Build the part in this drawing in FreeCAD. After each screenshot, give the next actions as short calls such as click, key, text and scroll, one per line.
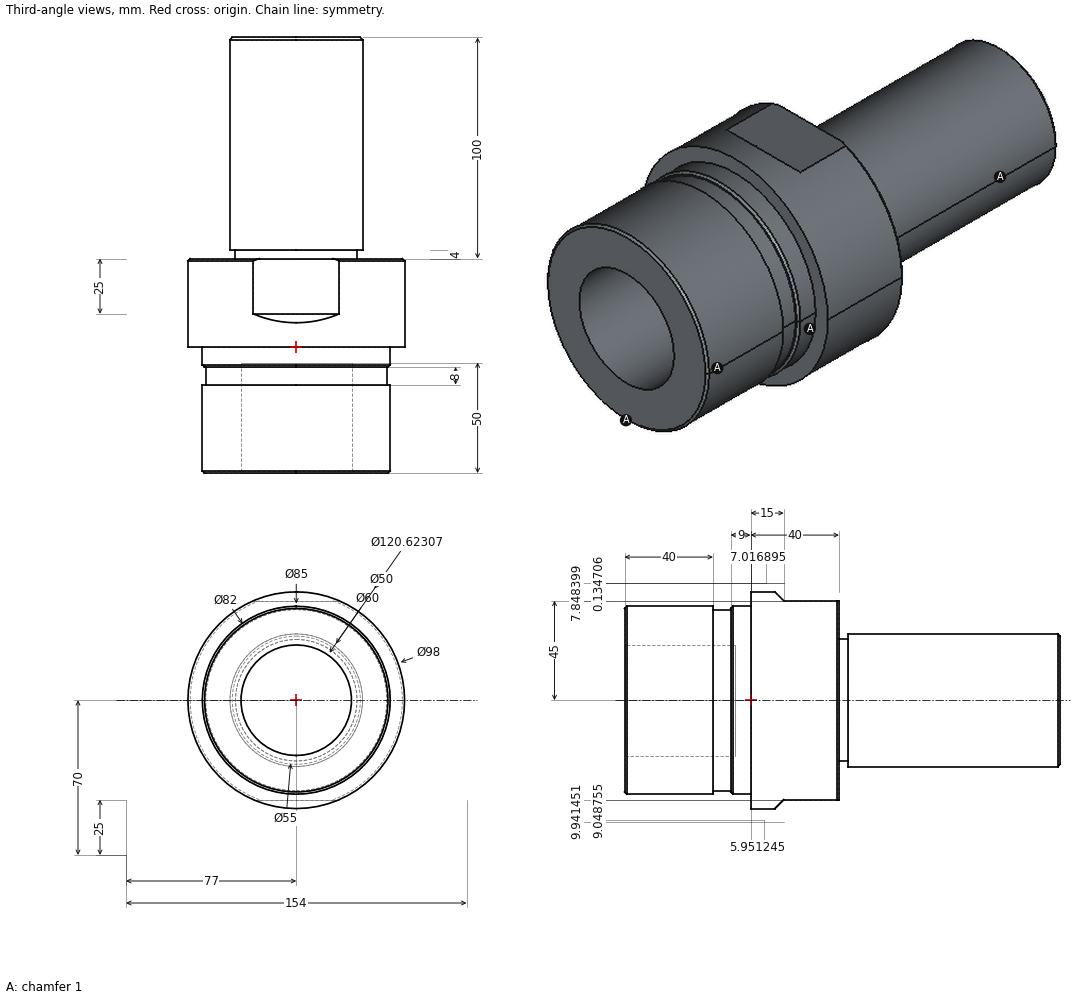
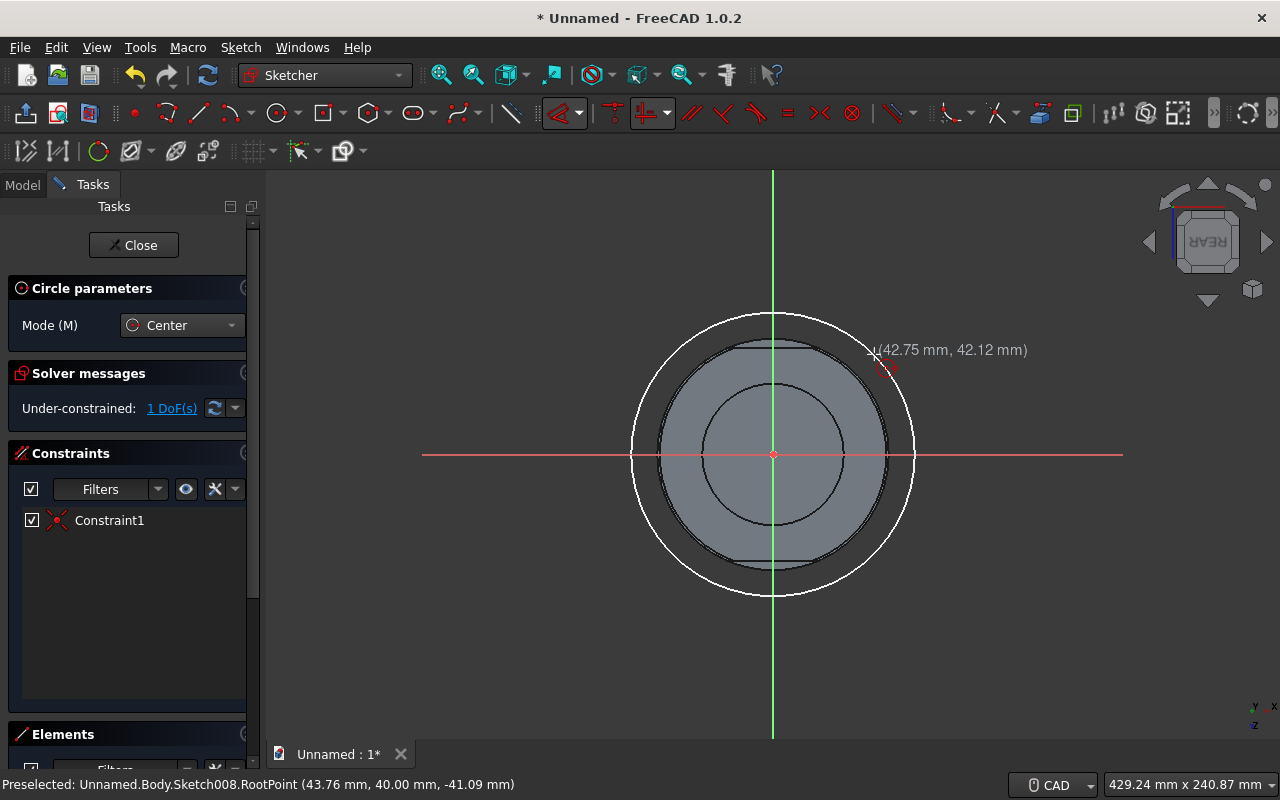
click(773, 454)
click(819, 409)
key(Escape)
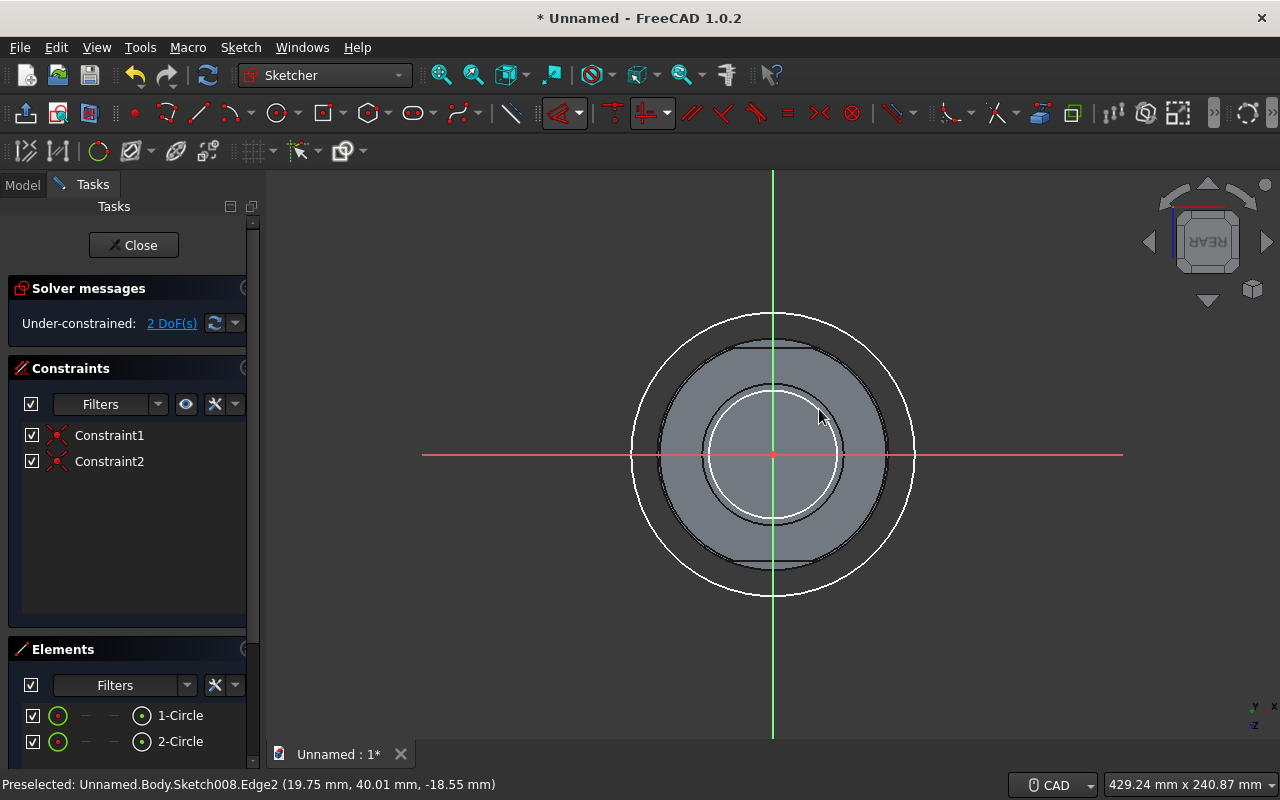
click(873, 354)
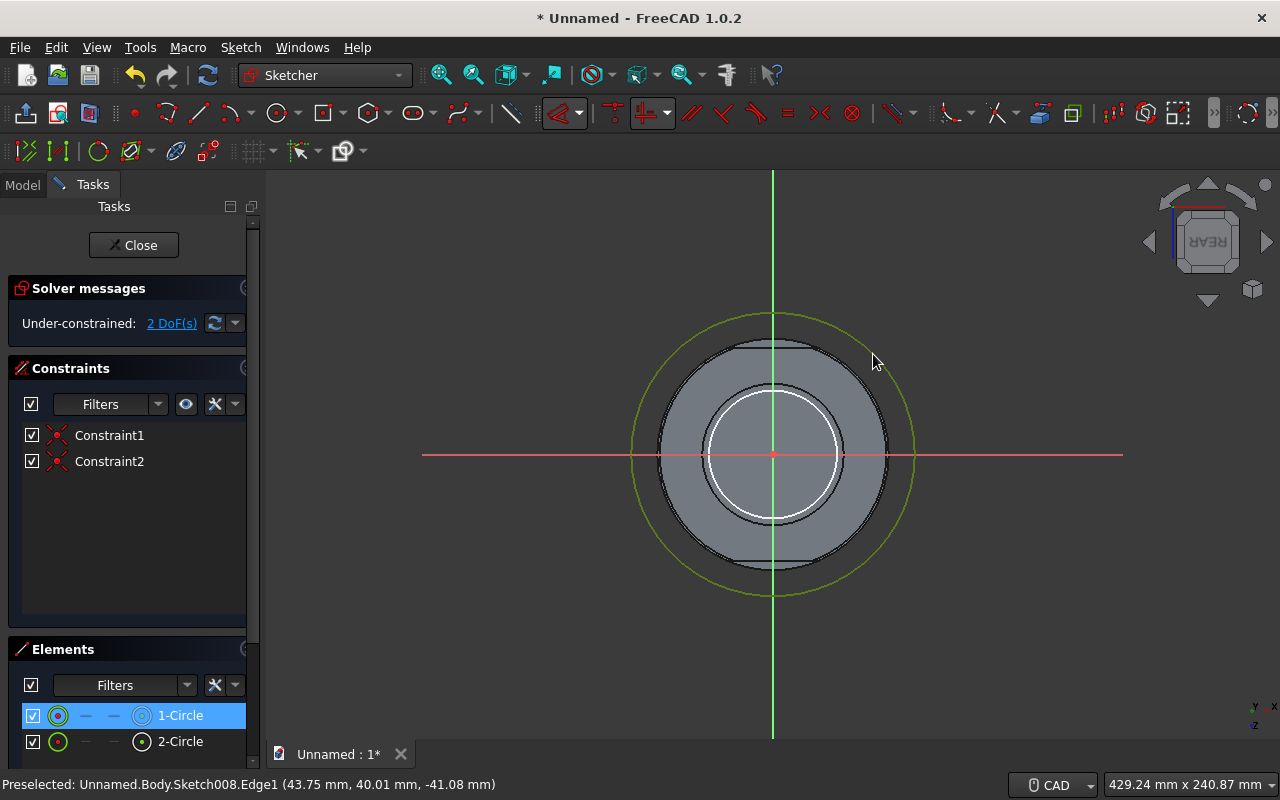
click(582, 114)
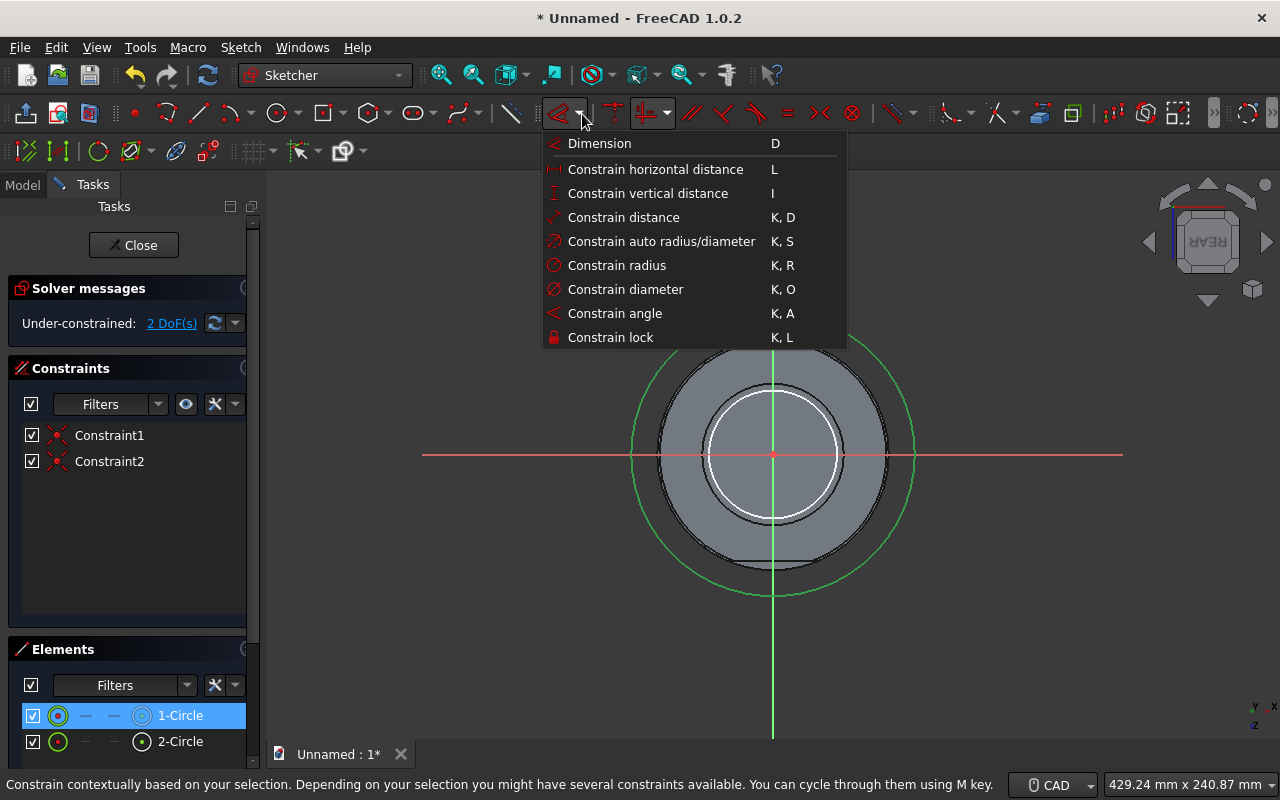
click(695, 289)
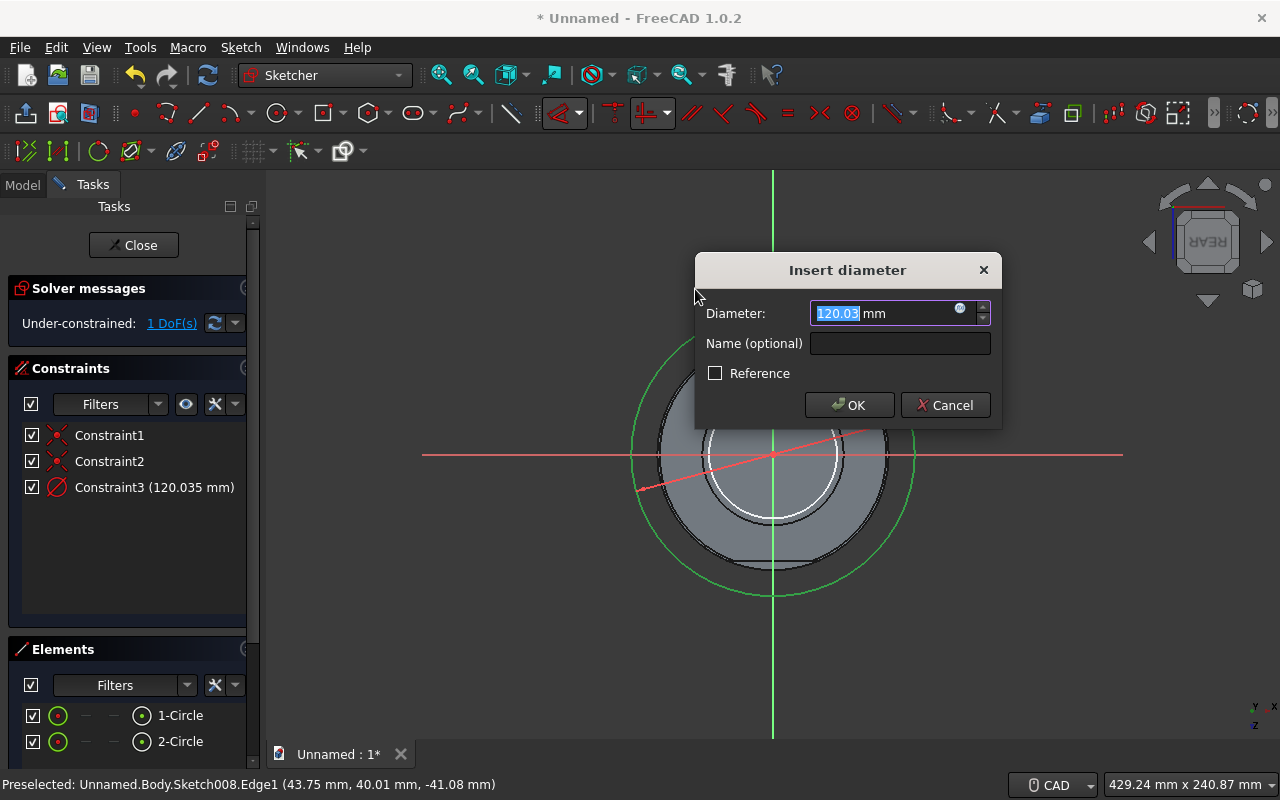
text(120.62307)
key(Return)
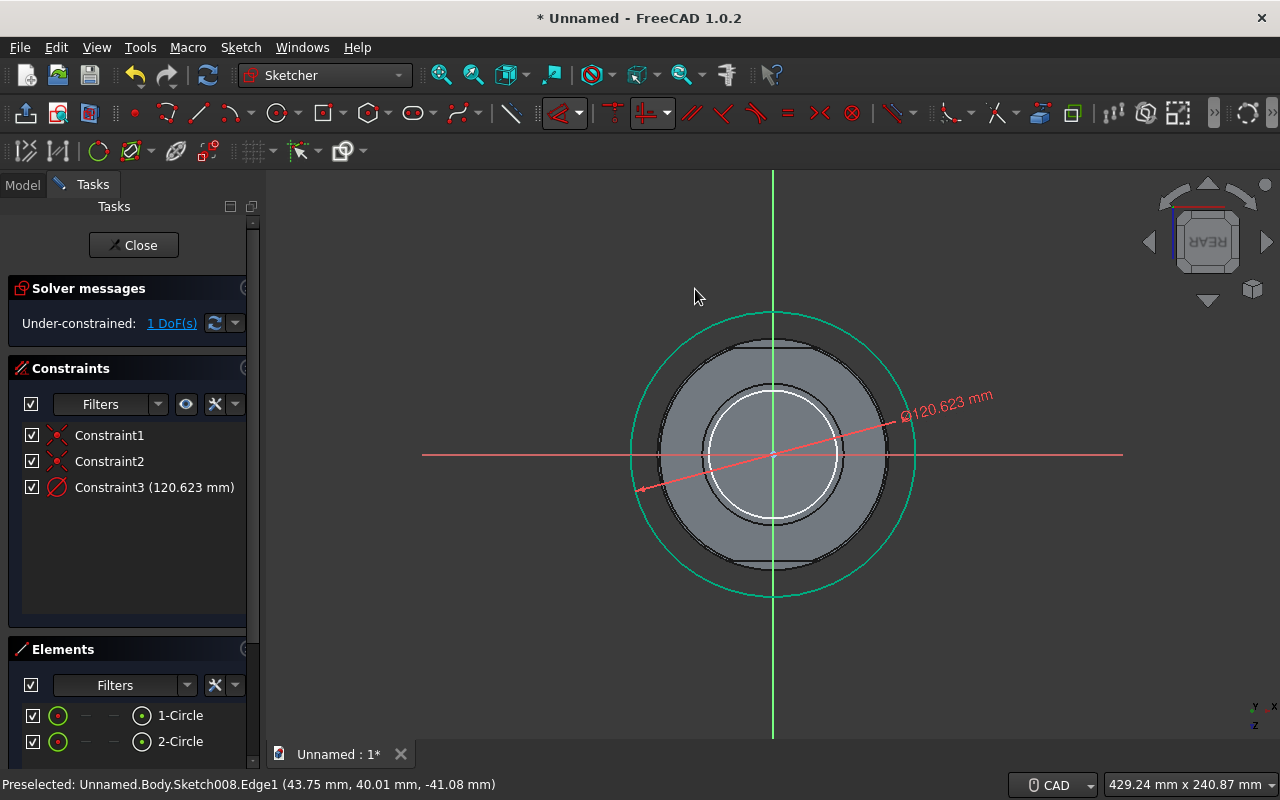
click(818, 409)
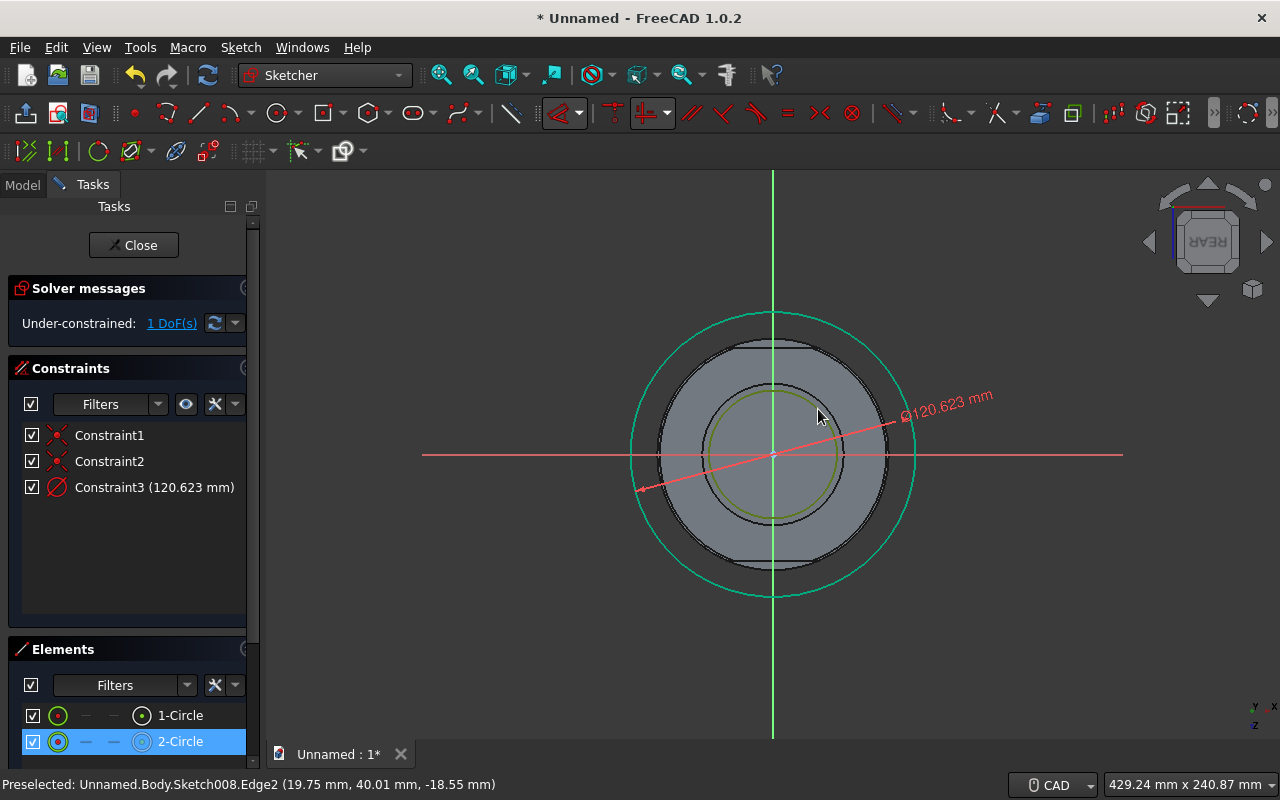
click(582, 114)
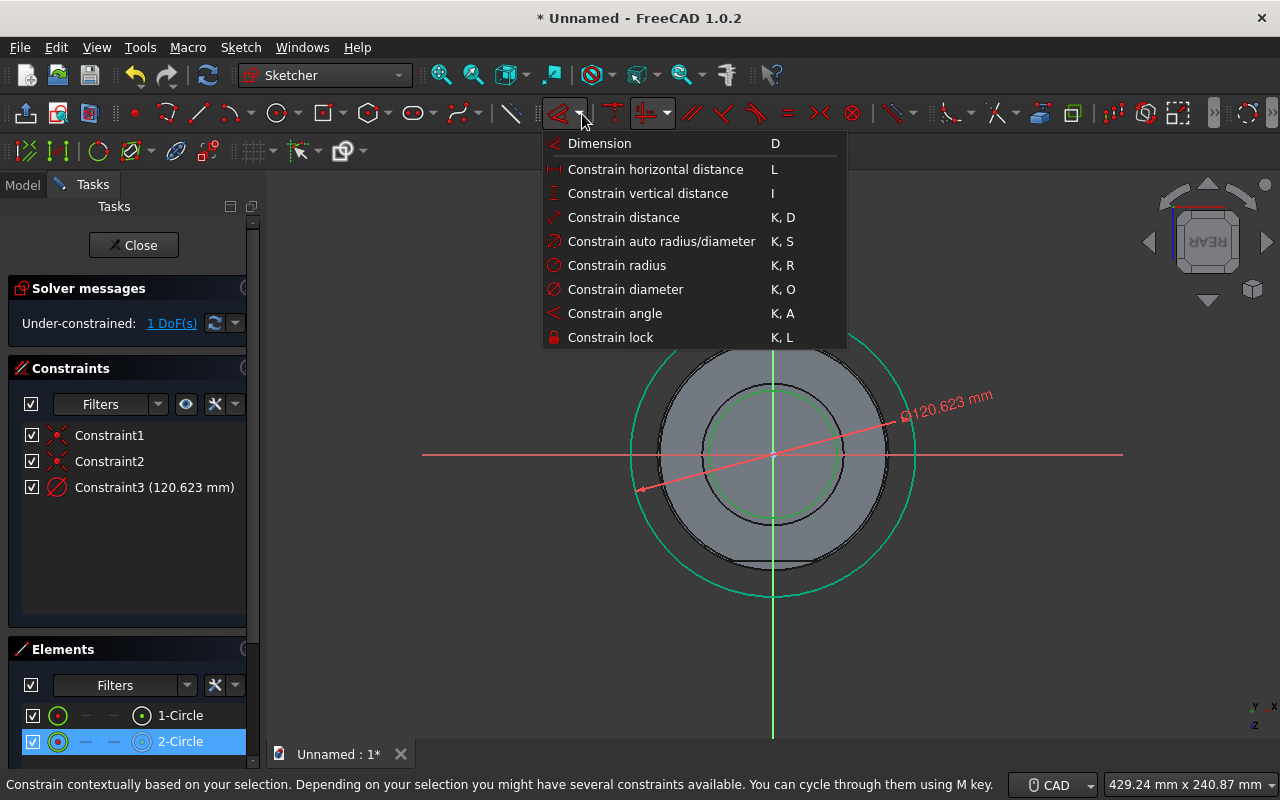
click(695, 289)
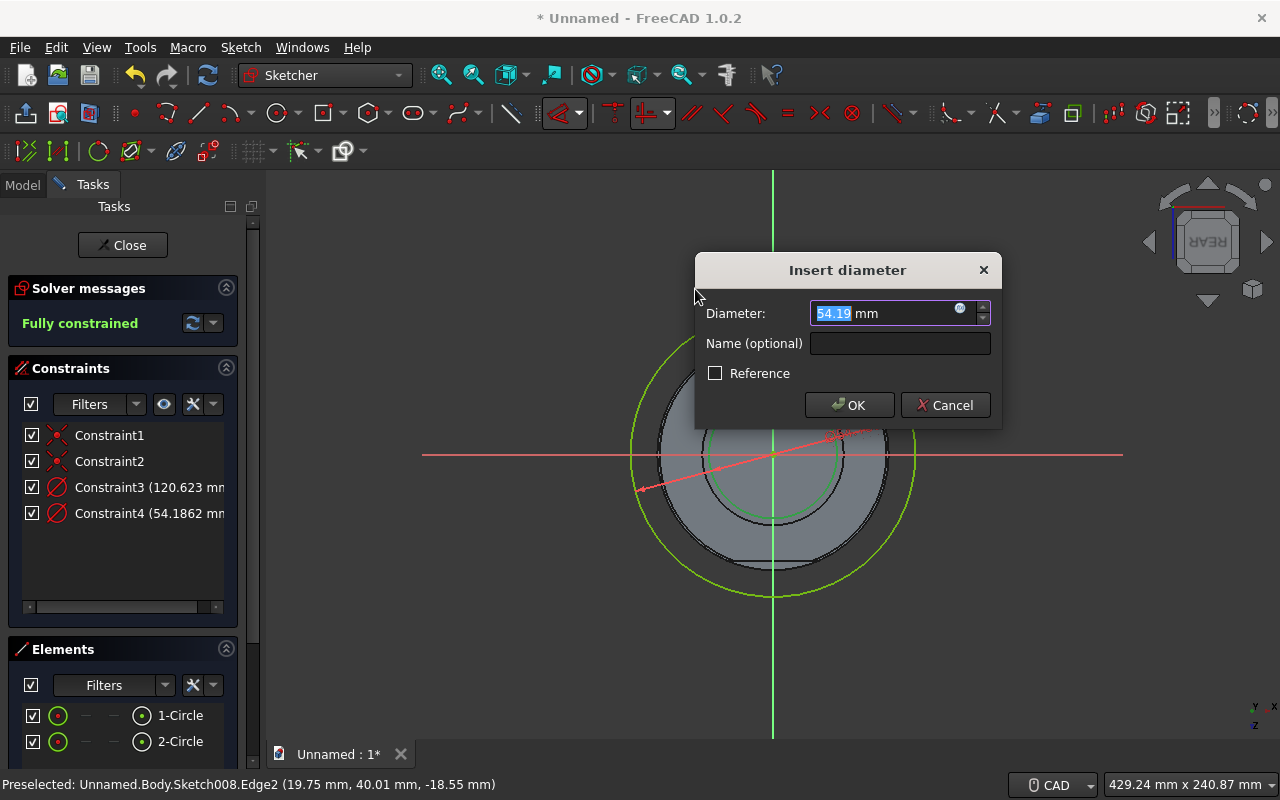
text(55)
key(Return)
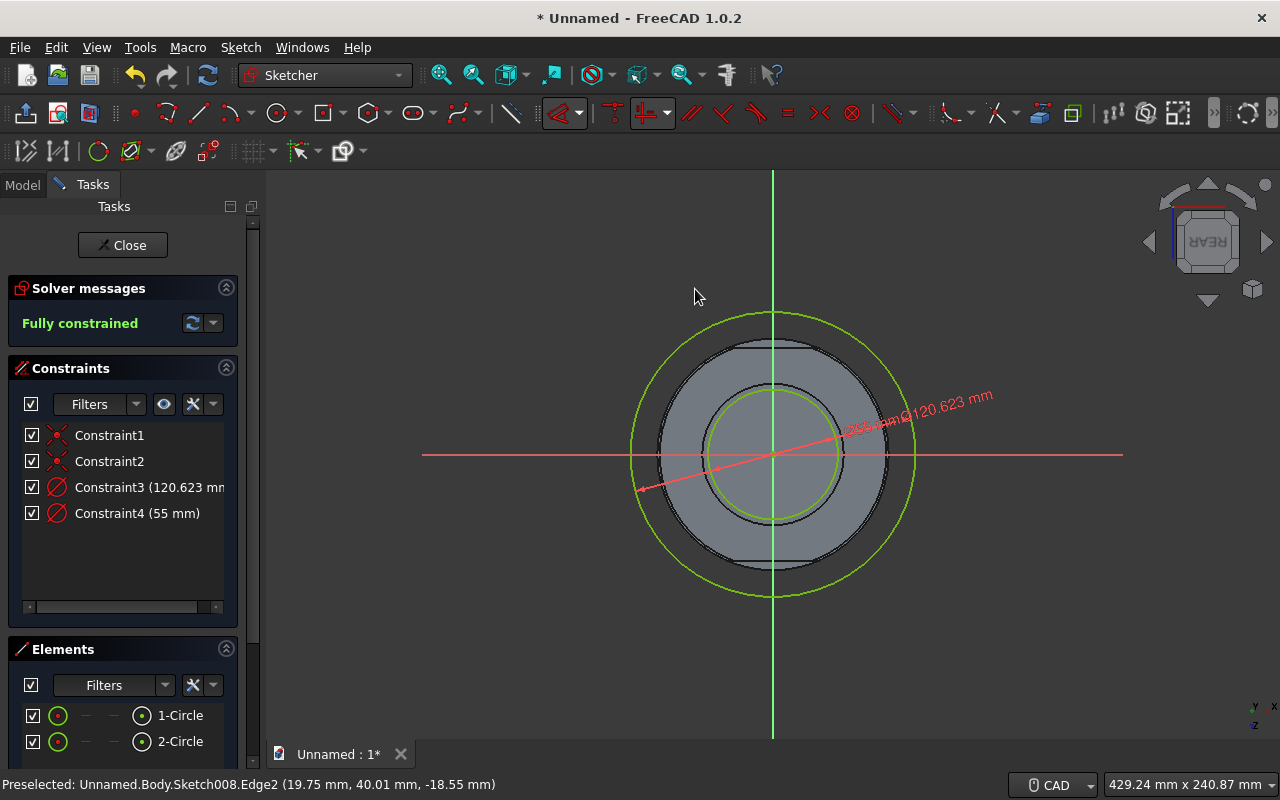
click(123, 245)